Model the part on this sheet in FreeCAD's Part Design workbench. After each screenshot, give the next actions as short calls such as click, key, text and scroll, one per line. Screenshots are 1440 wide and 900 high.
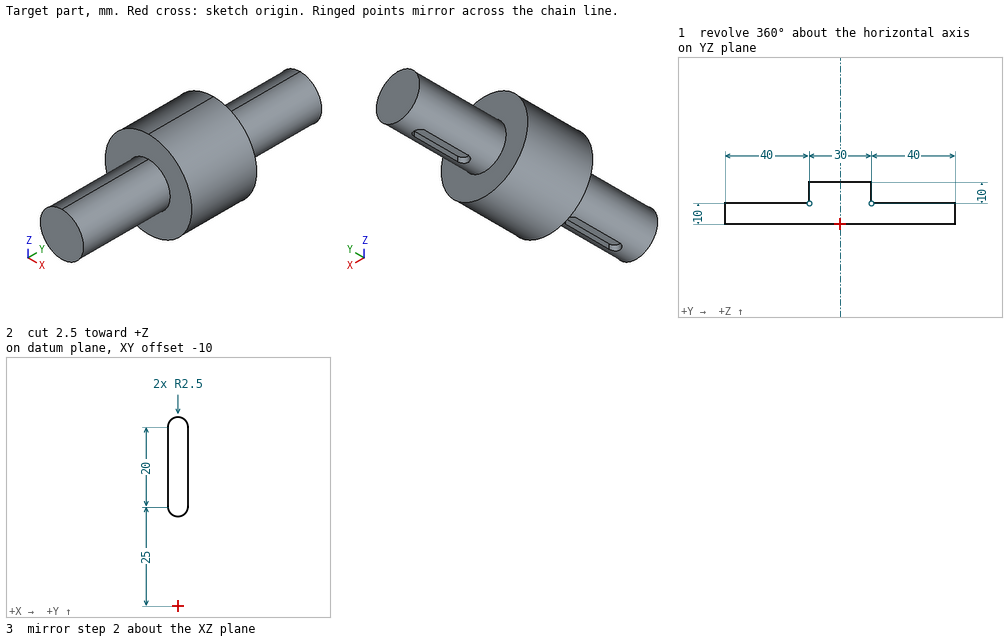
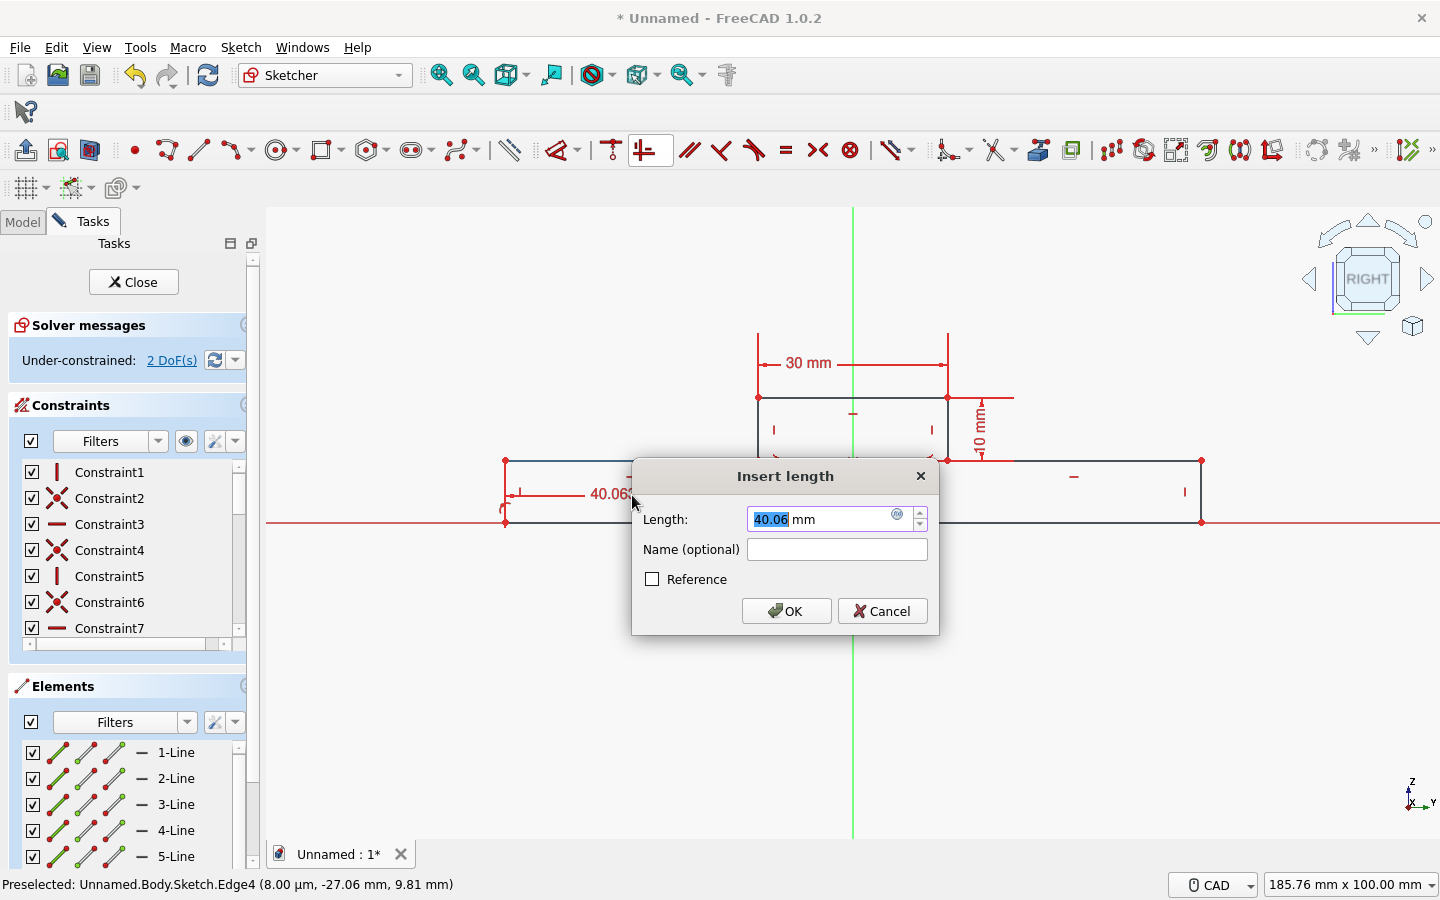
text(40)
key(Return)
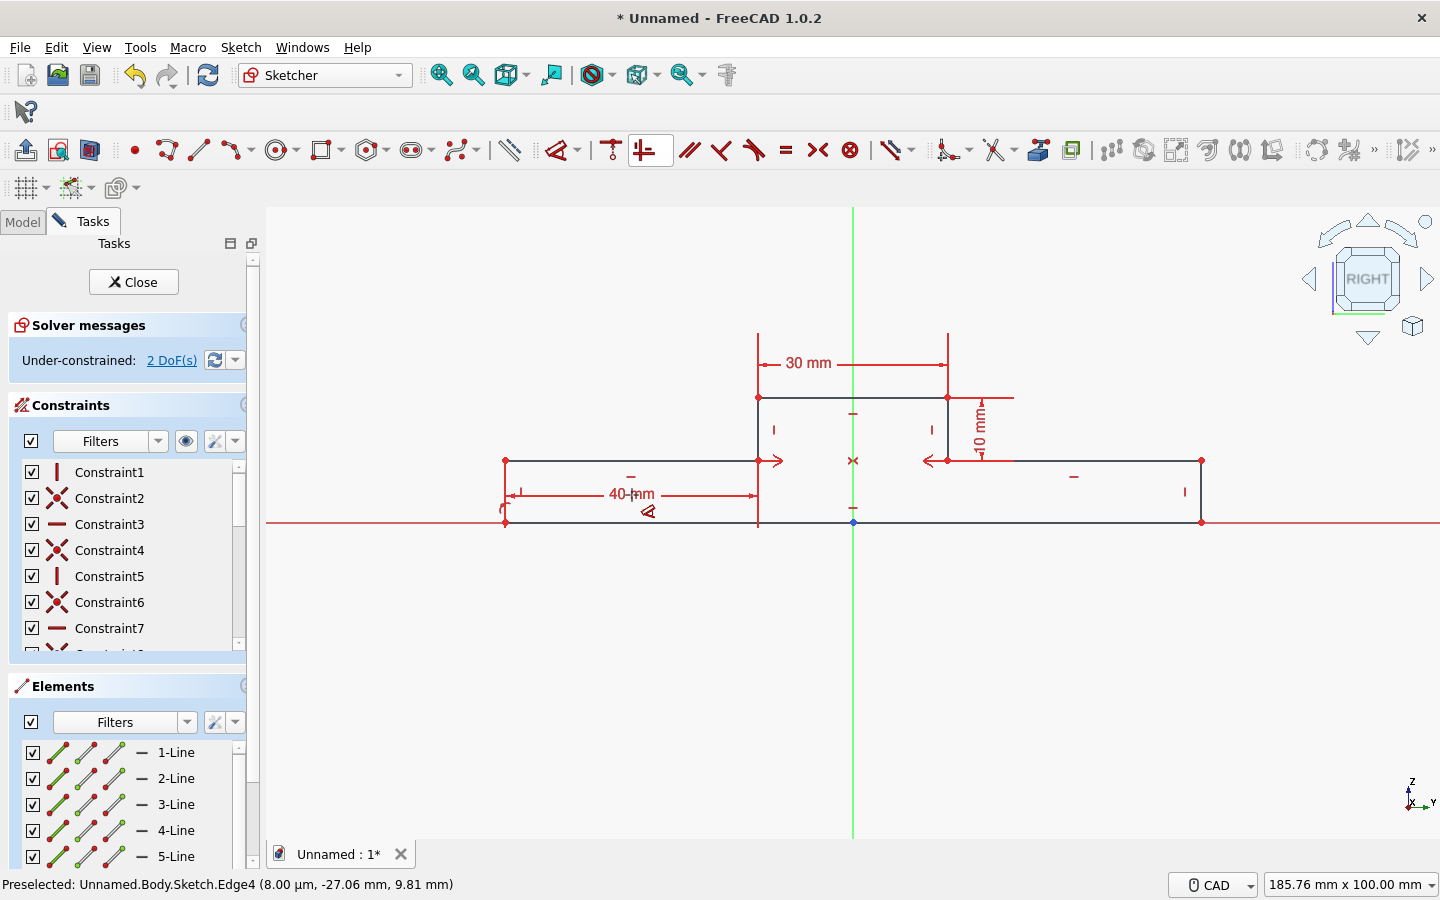
click(505, 480)
click(471, 492)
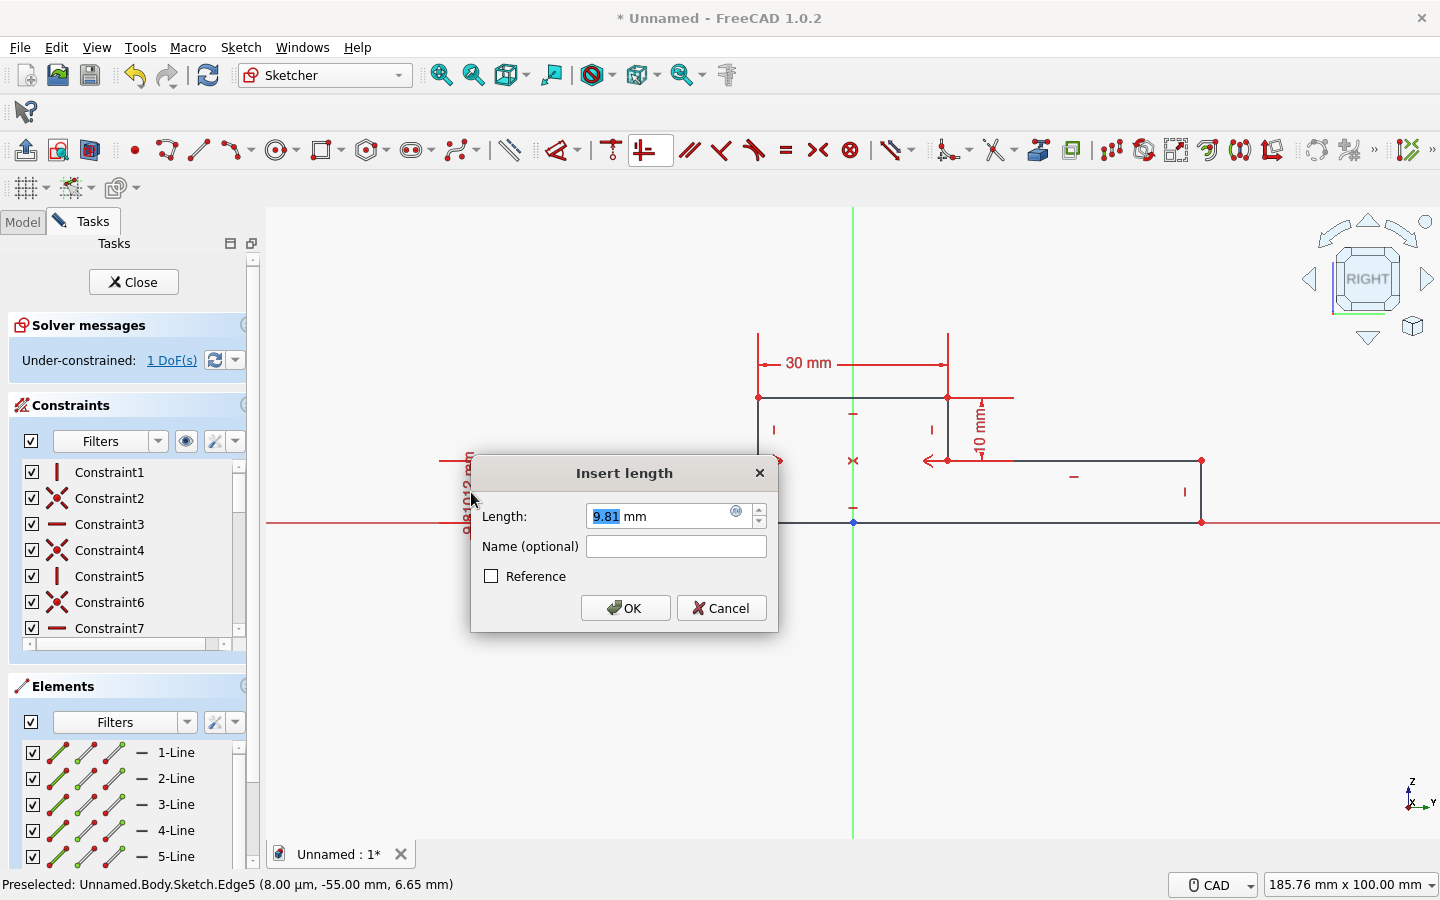
text(10)
key(Return)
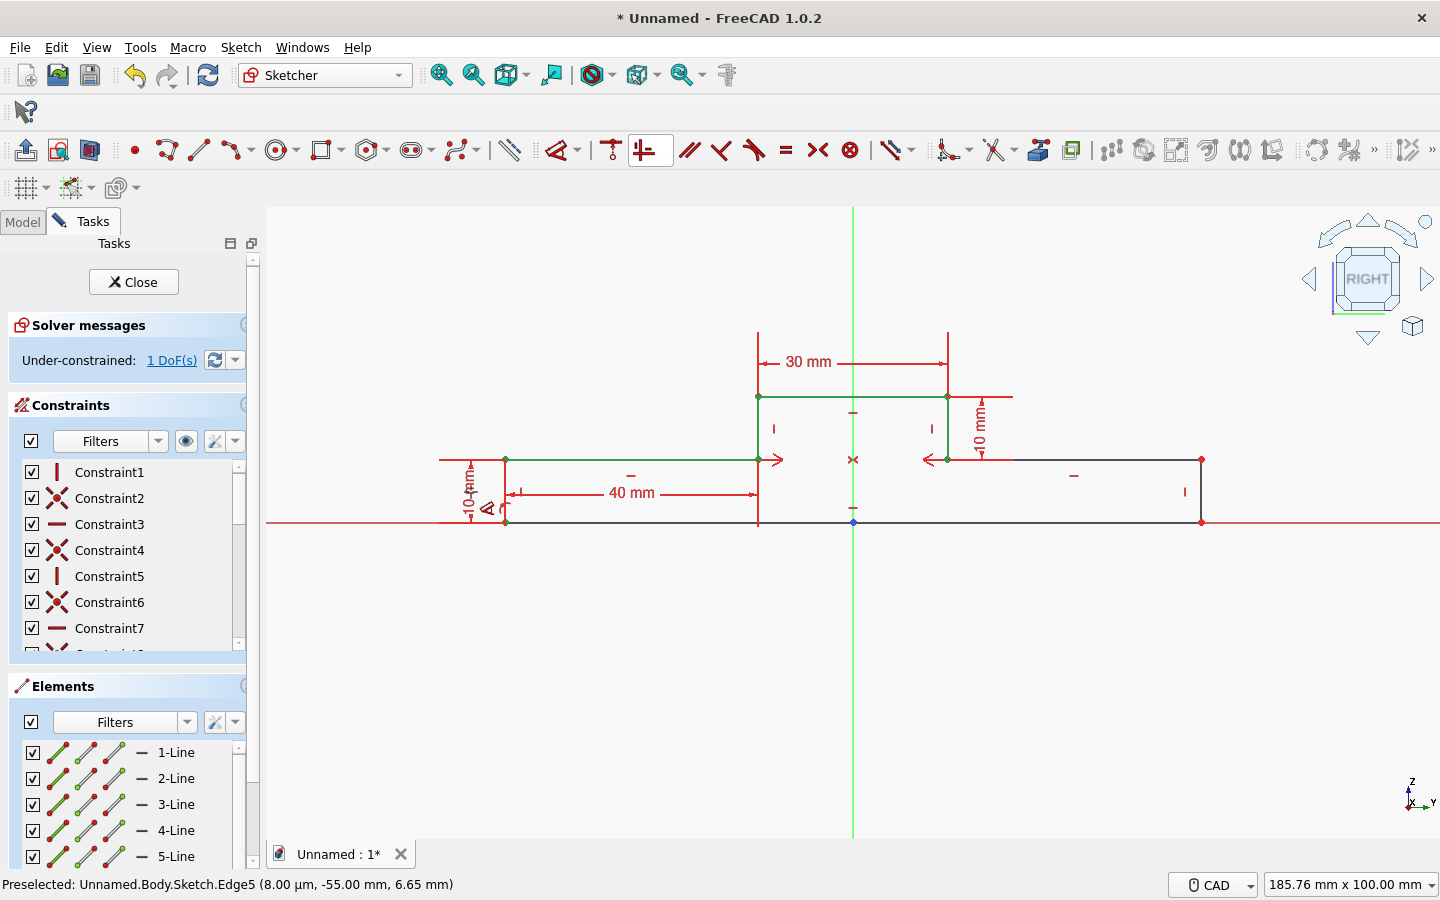
click(1125, 460)
click(1074, 494)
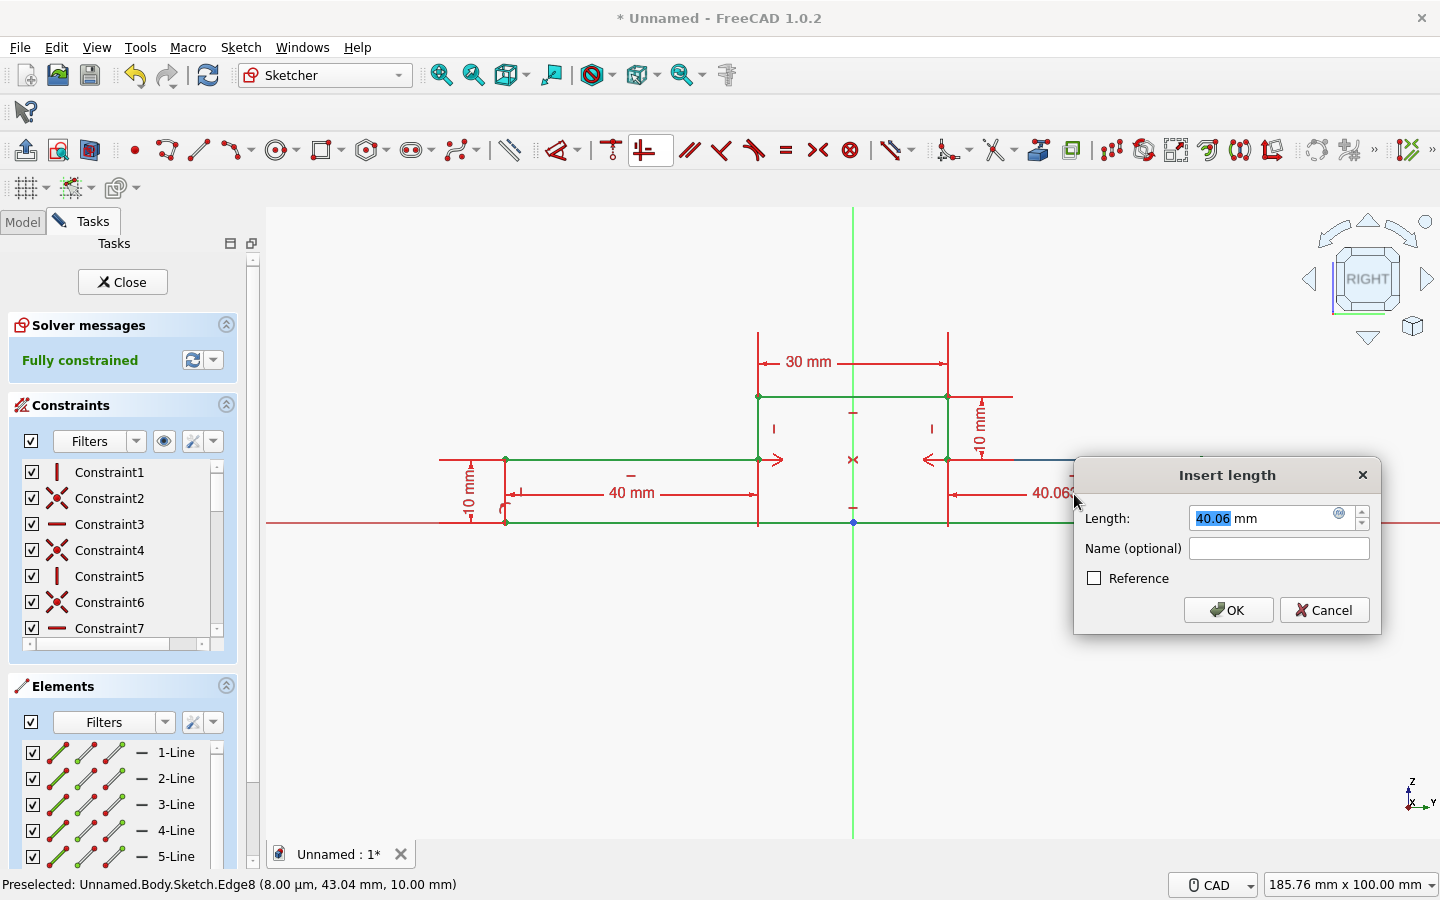
text(40)
key(Return)
key(Escape)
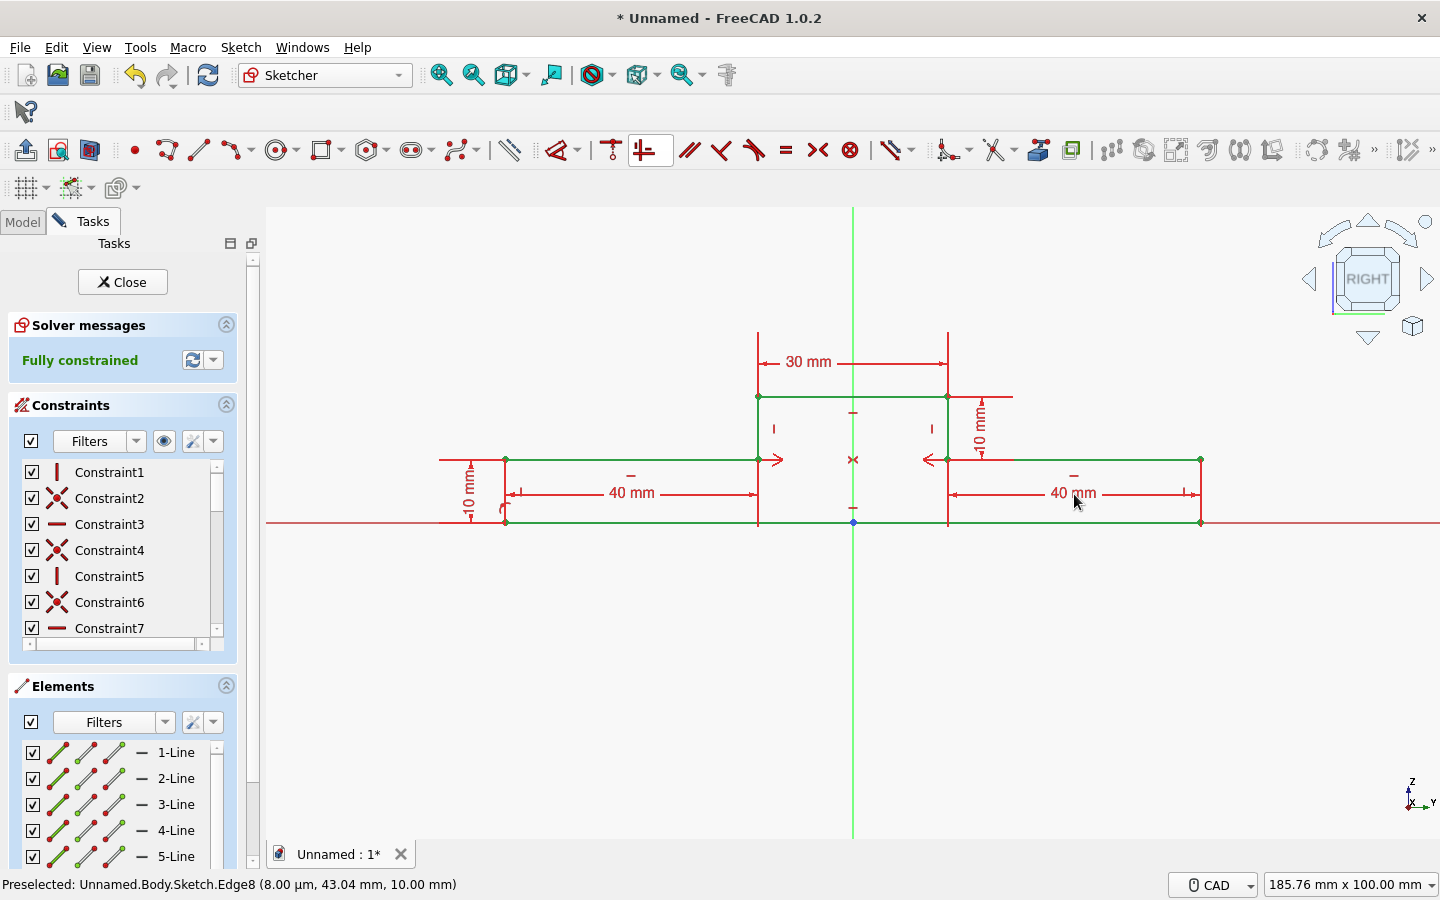
click(123, 282)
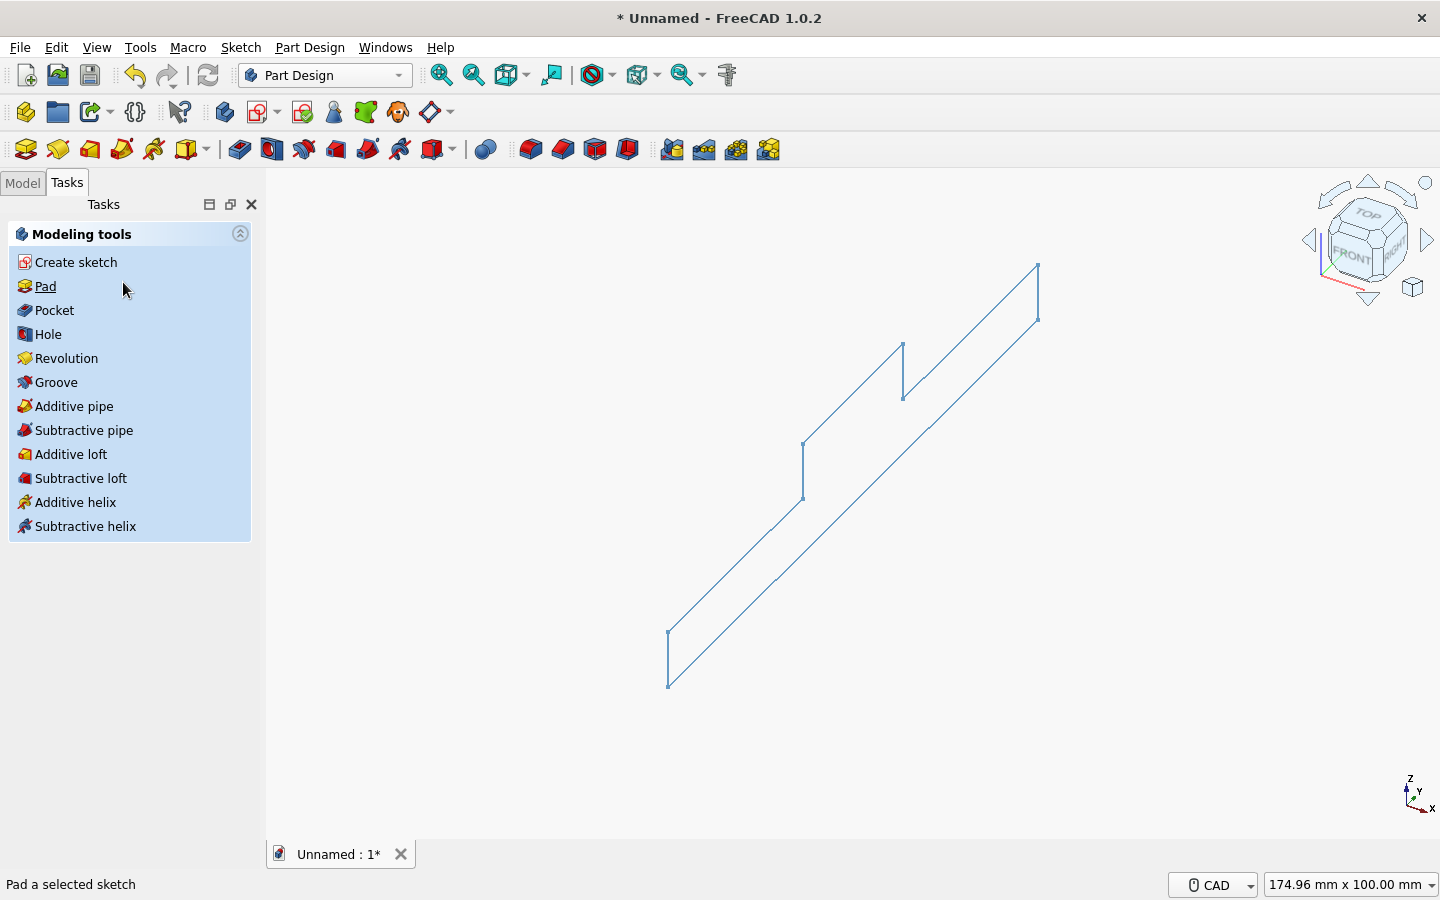
click(58, 150)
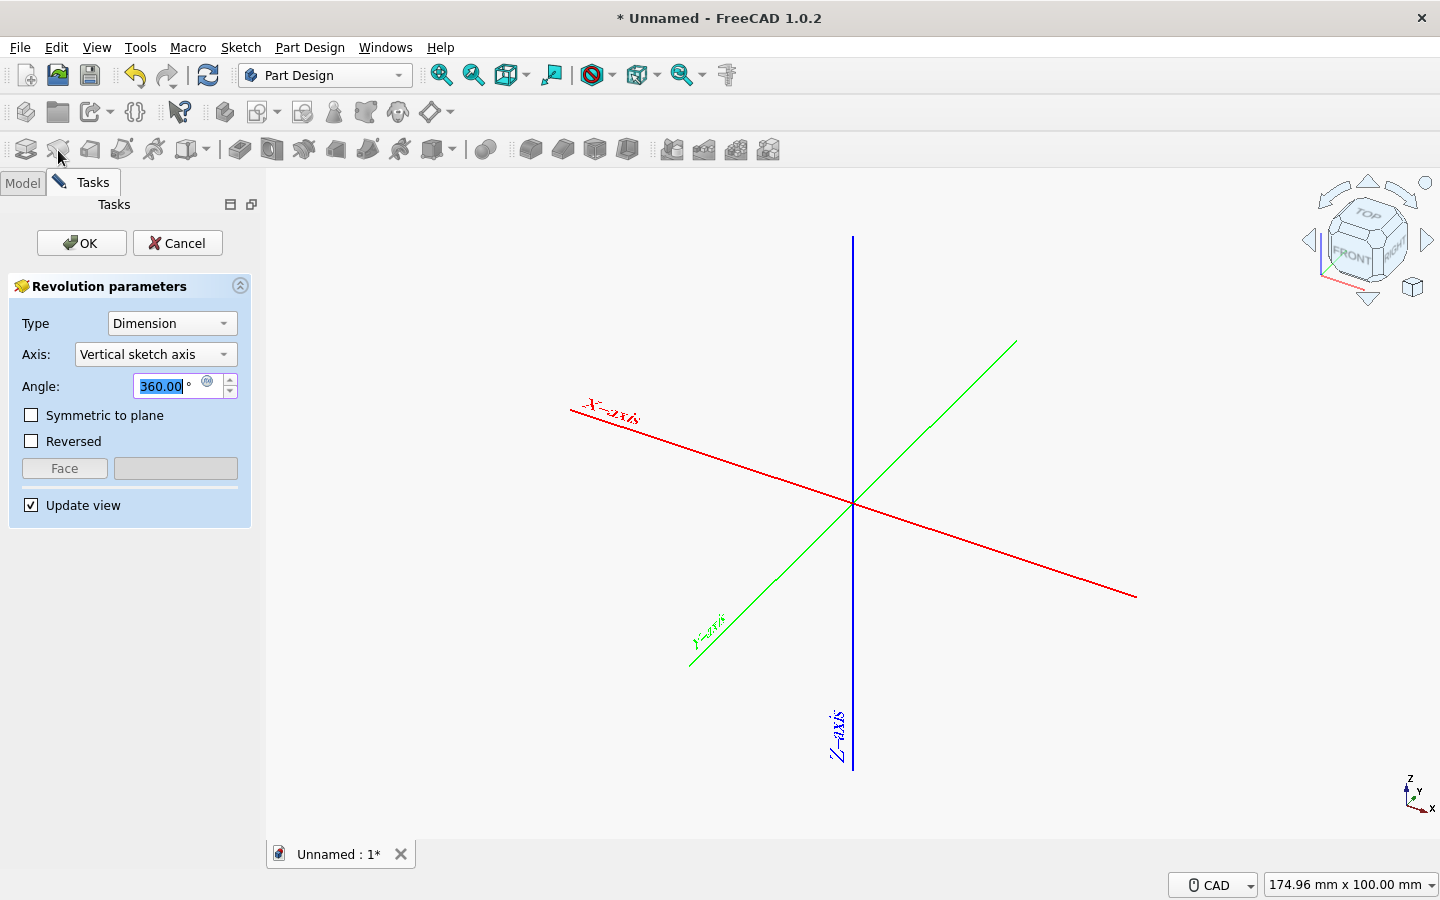
click(156, 354)